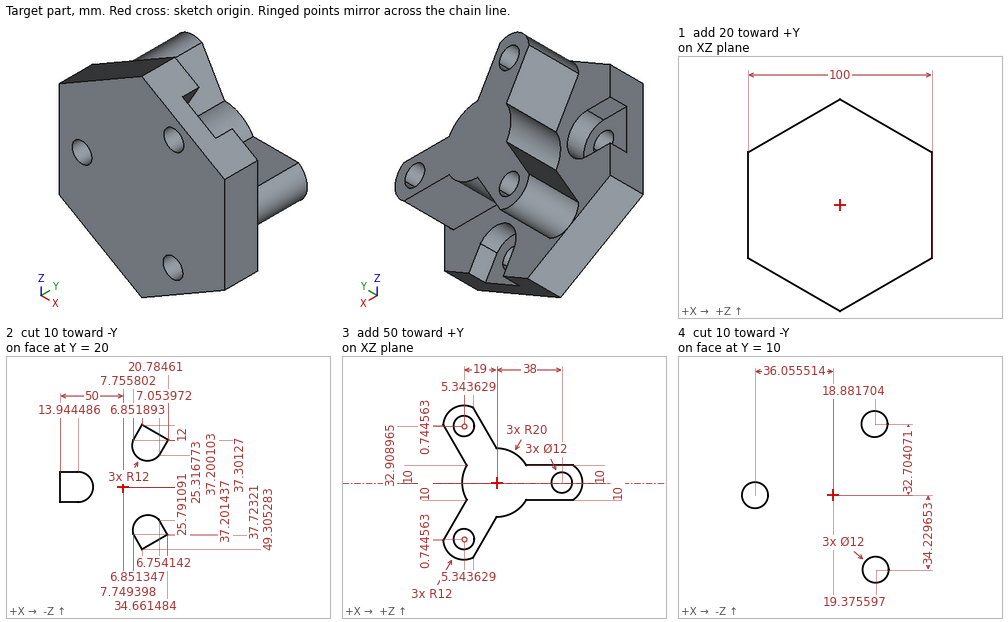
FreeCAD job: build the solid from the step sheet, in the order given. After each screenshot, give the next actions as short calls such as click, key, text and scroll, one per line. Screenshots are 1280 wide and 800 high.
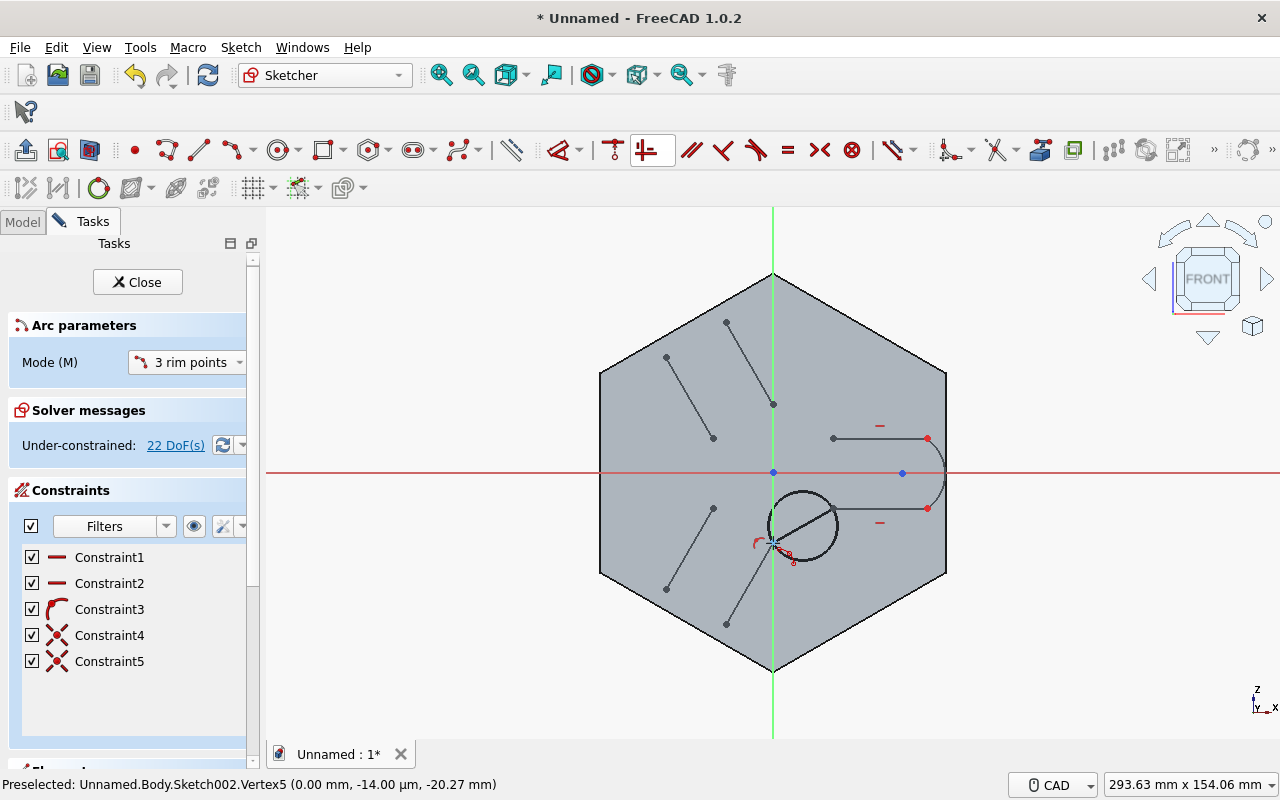
scroll(808, 533, up, 3)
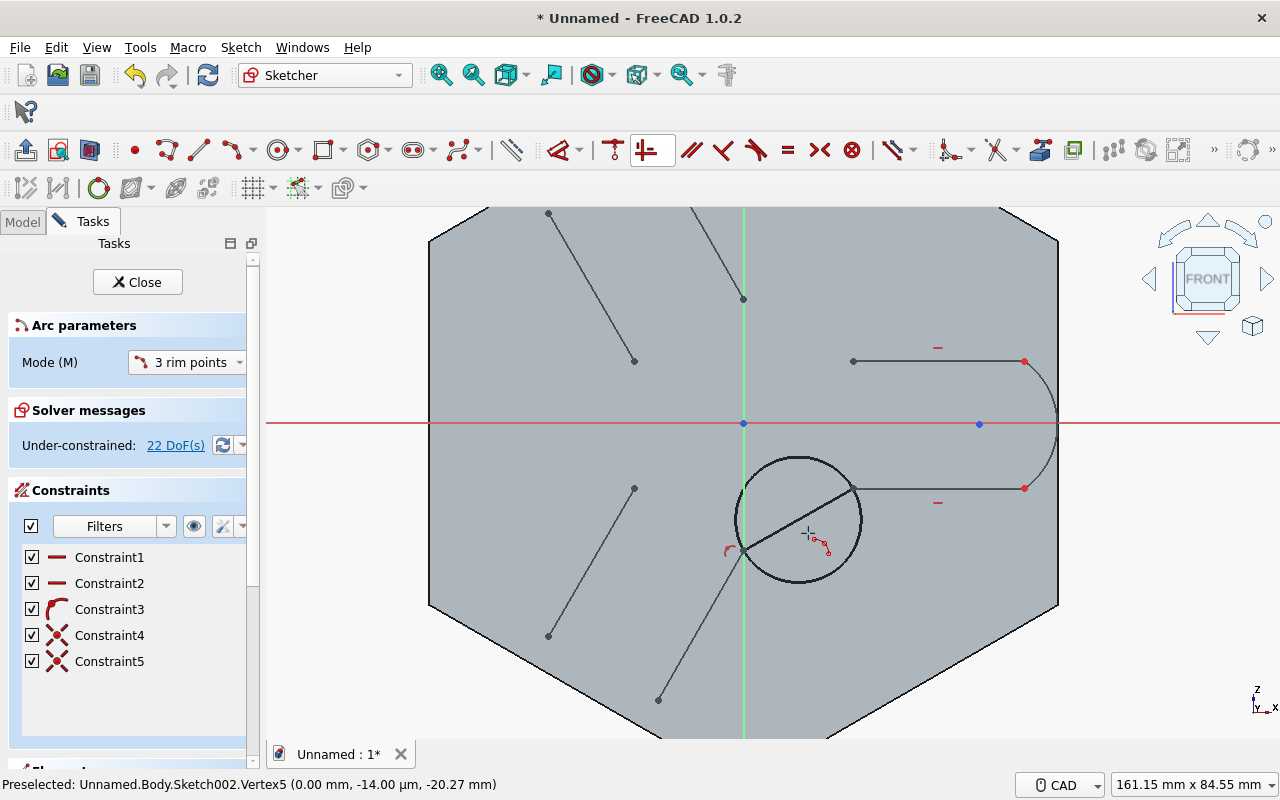
click(807, 532)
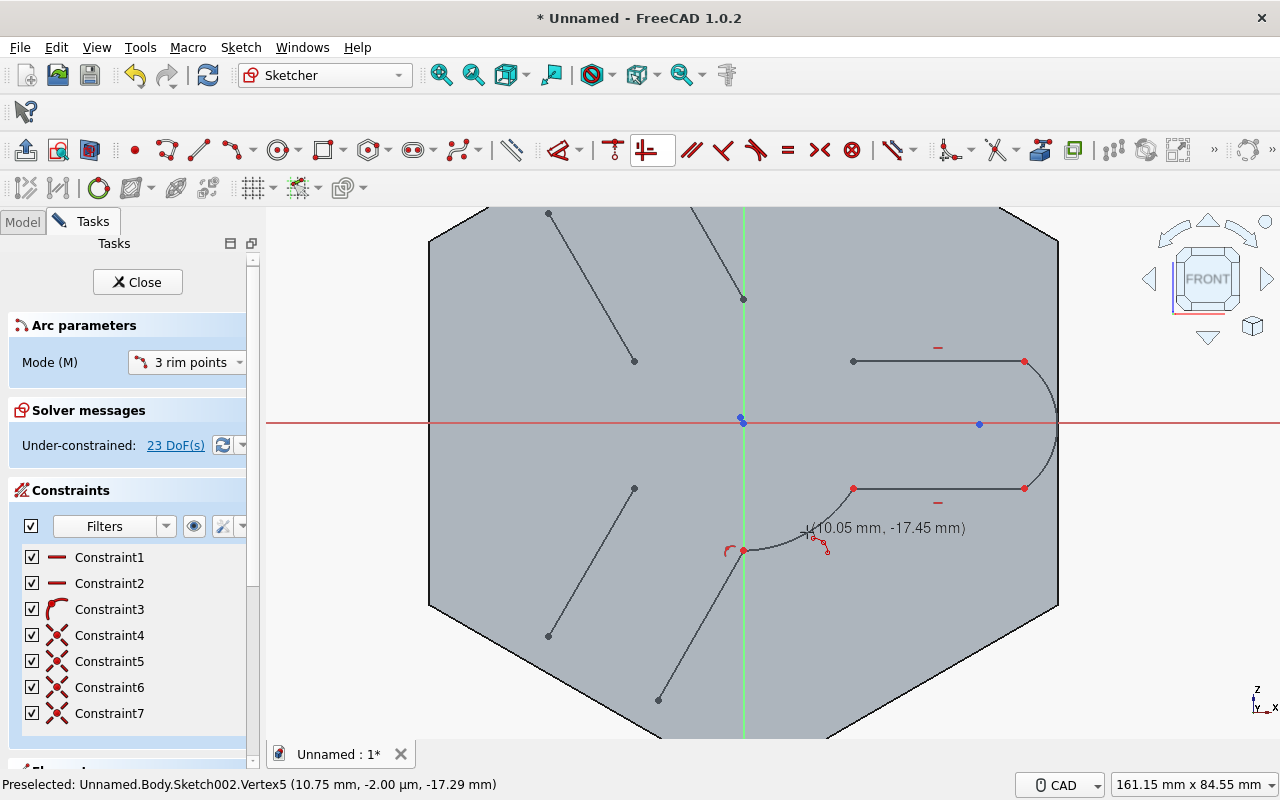
click(658, 700)
click(549, 636)
click(586, 696)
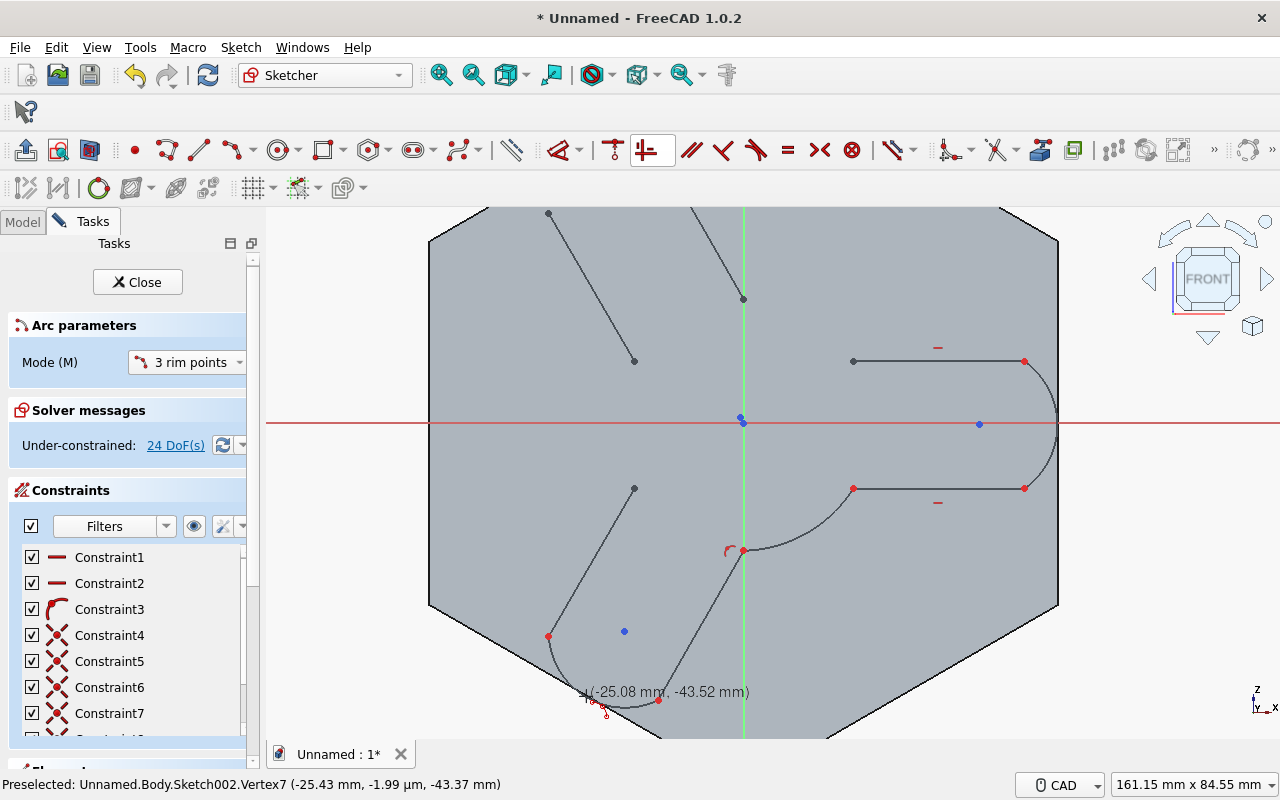
click(634, 489)
click(634, 361)
click(621, 397)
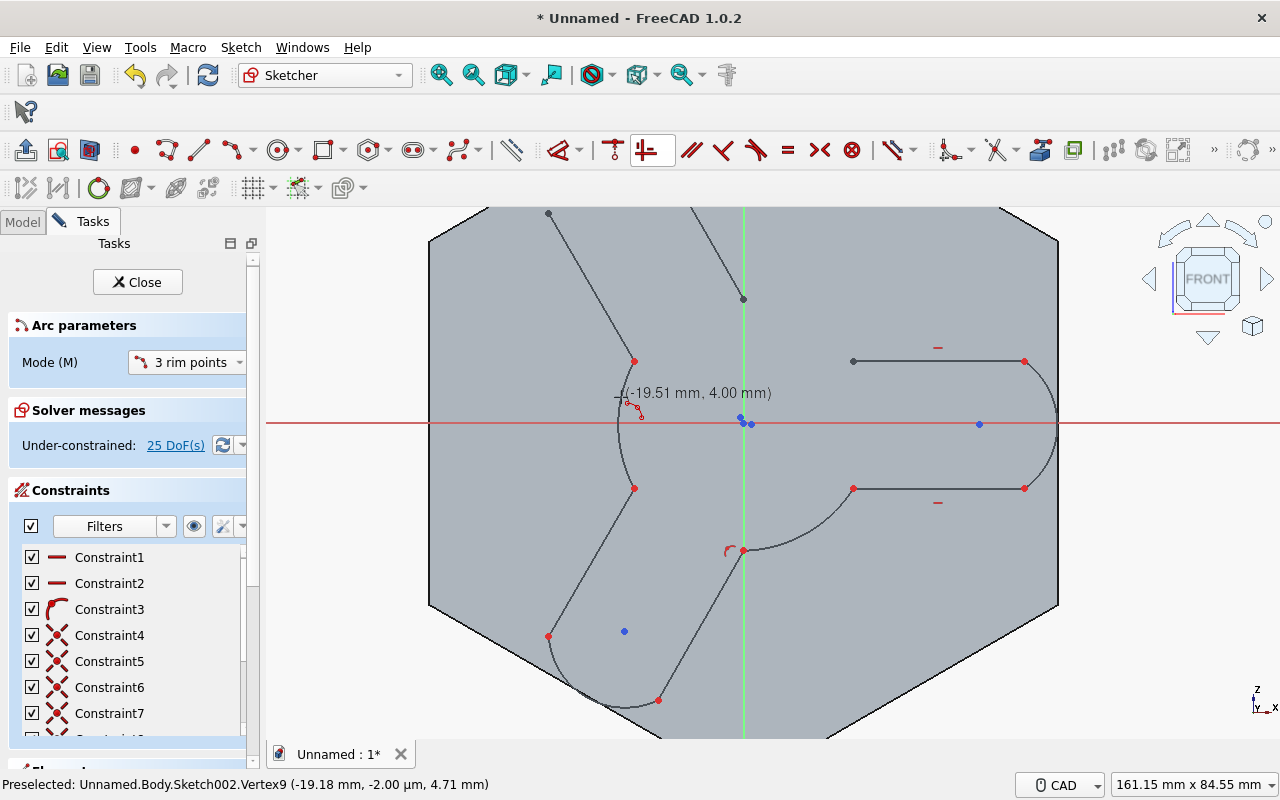
scroll(503, 574, down, 2)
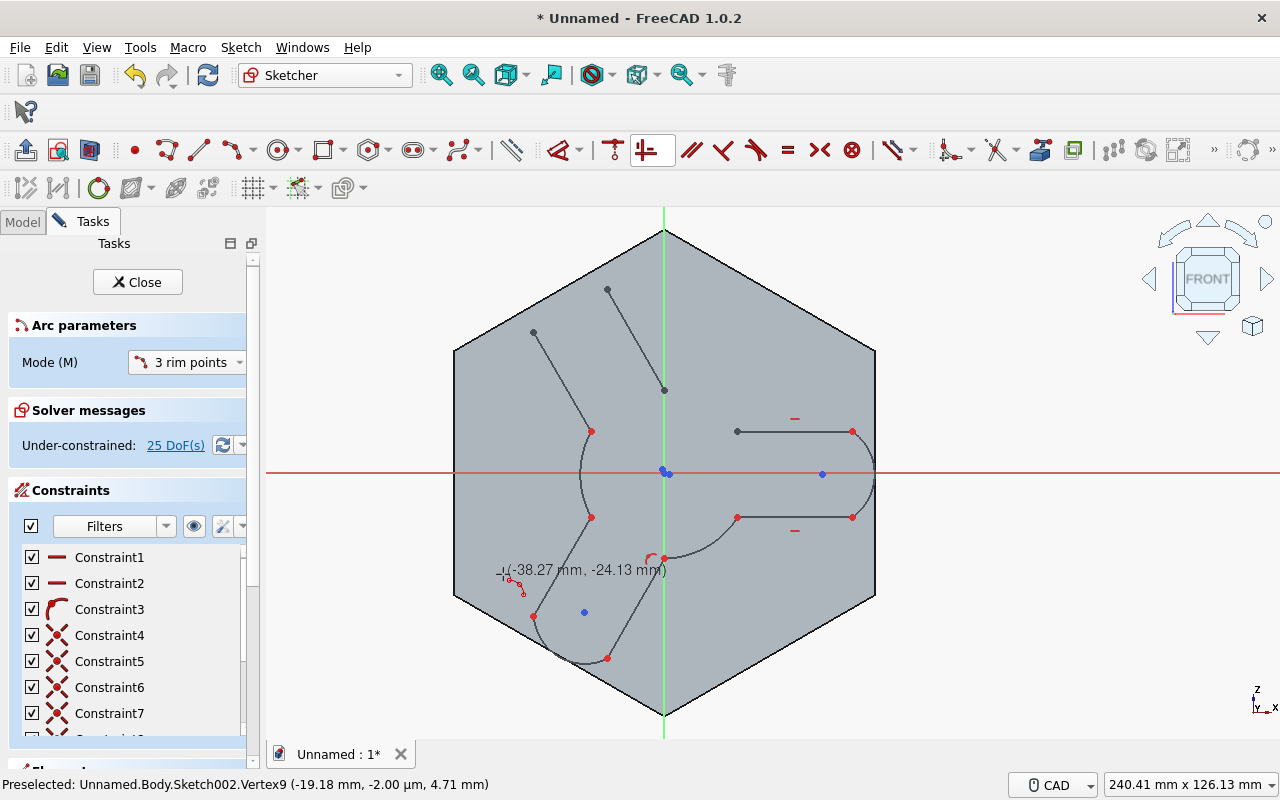
click(534, 333)
click(607, 290)
click(559, 290)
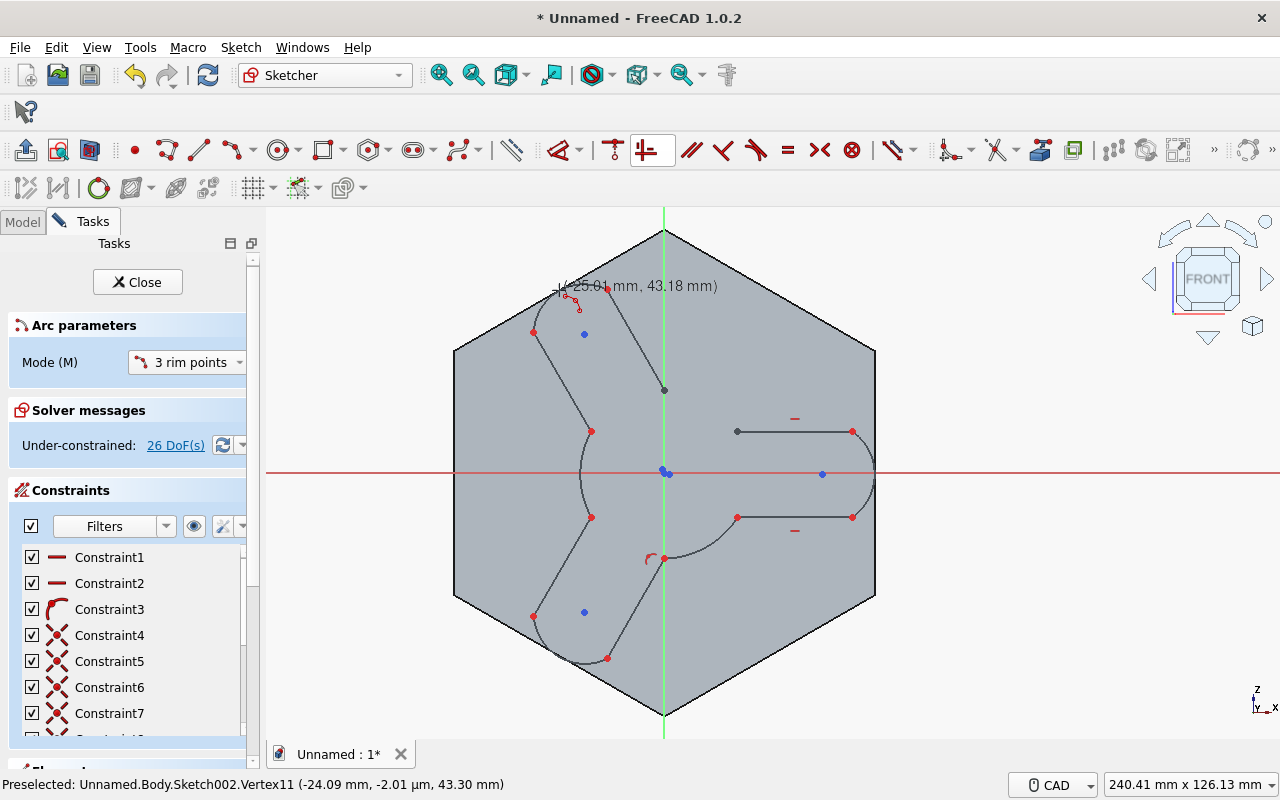
click(664, 390)
click(738, 432)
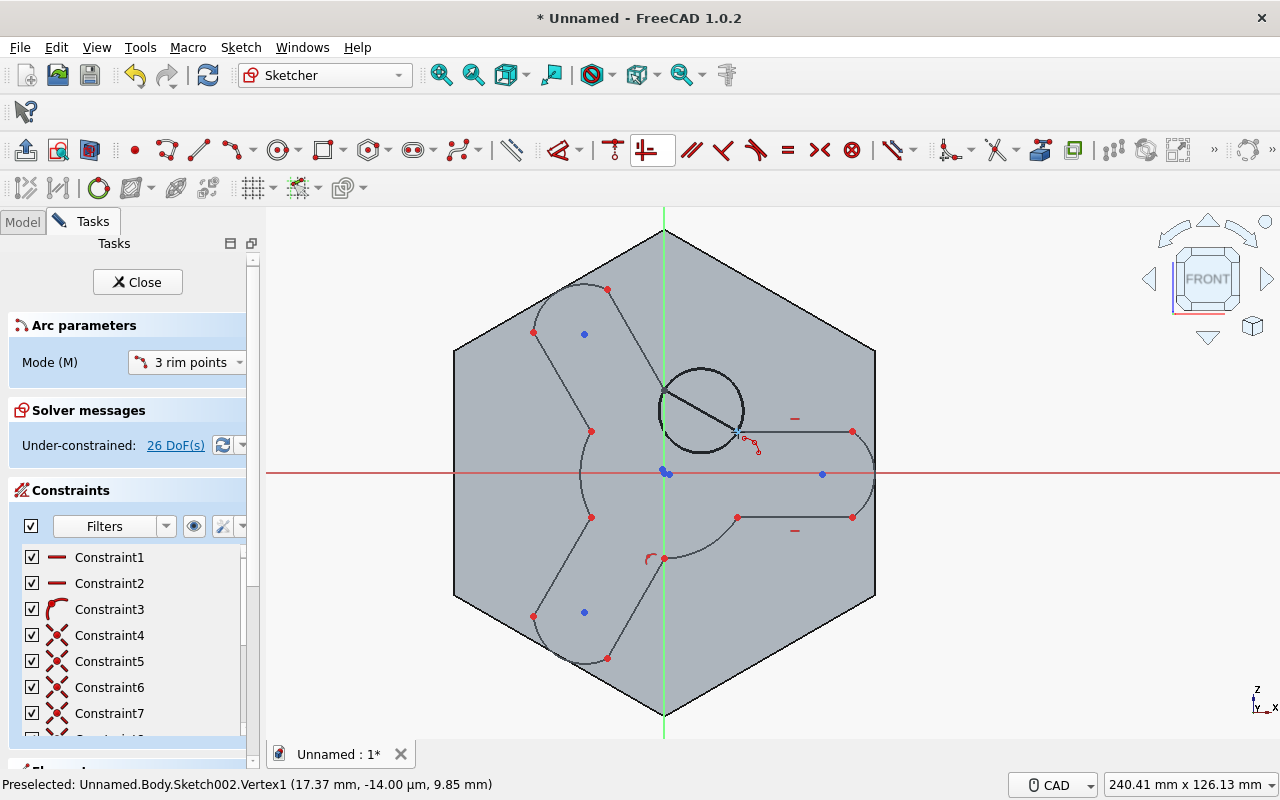
scroll(707, 400, up, 2)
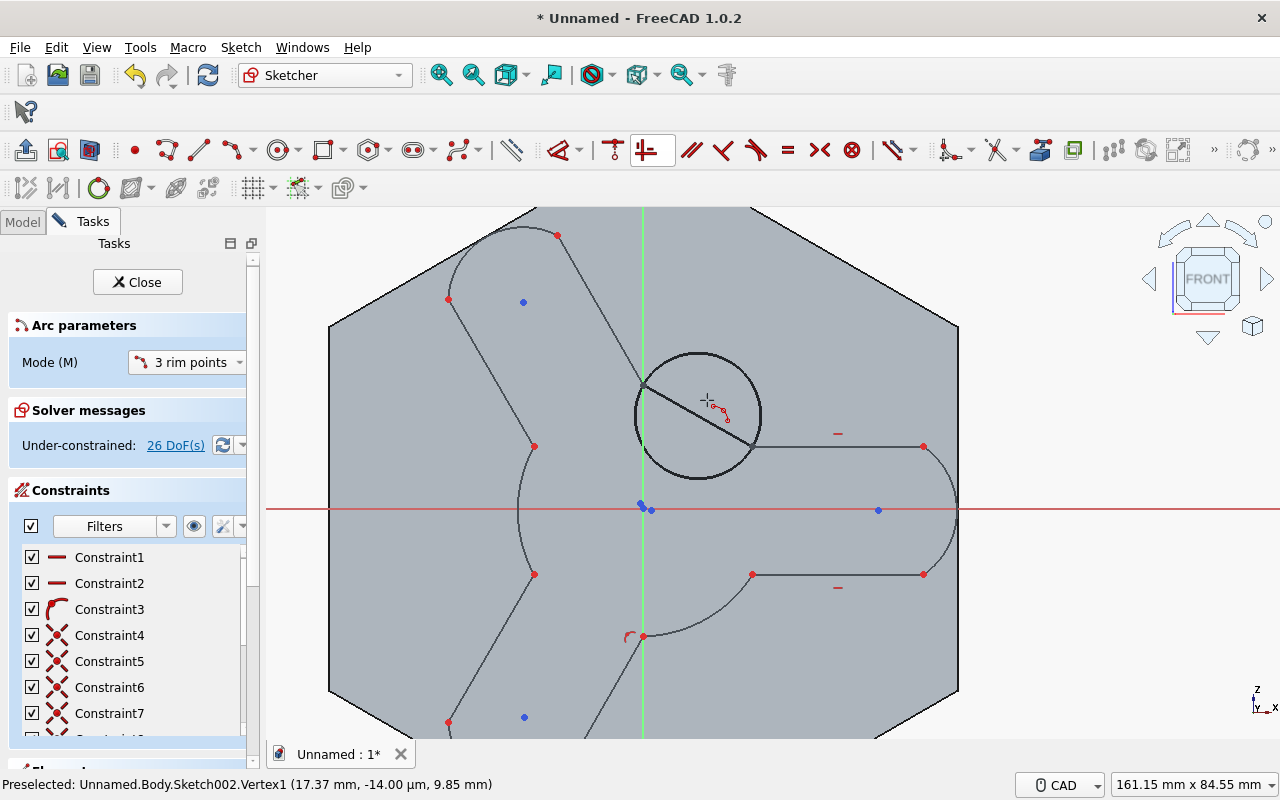
click(706, 400)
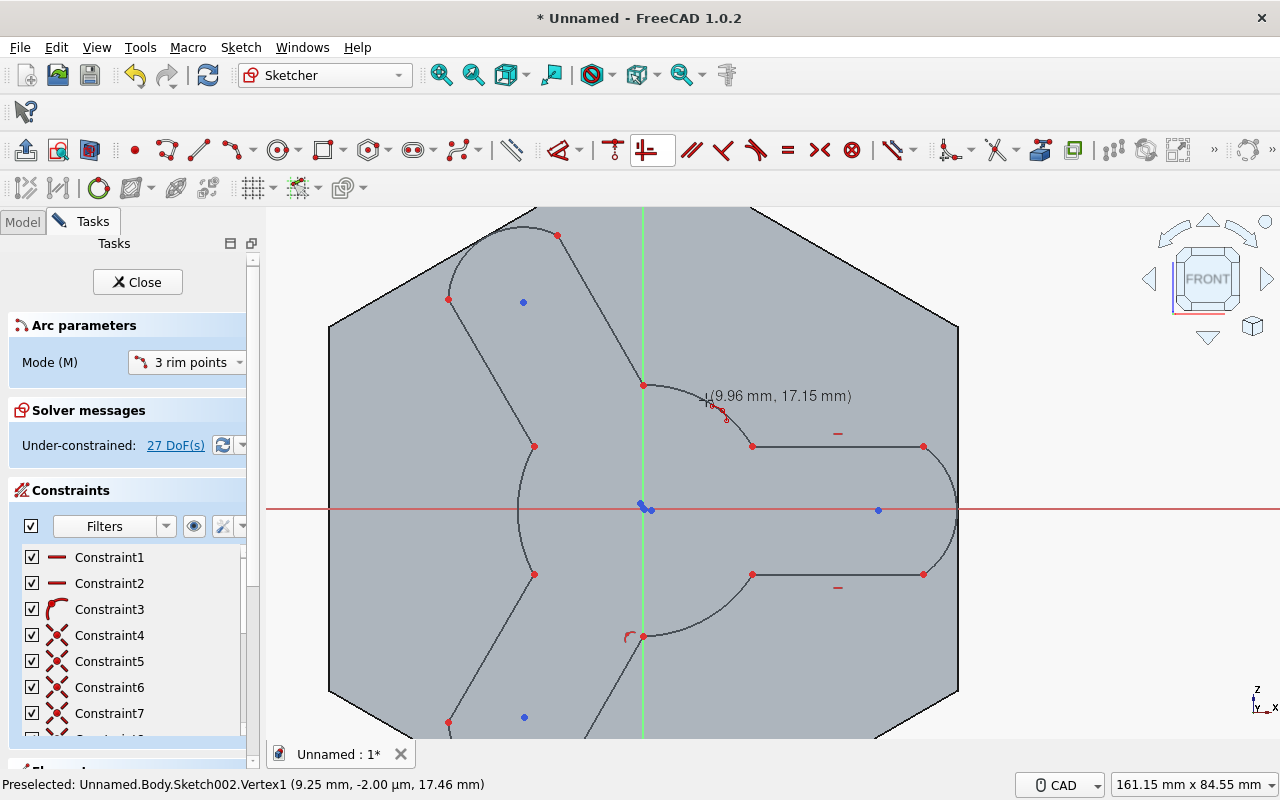
click(278, 150)